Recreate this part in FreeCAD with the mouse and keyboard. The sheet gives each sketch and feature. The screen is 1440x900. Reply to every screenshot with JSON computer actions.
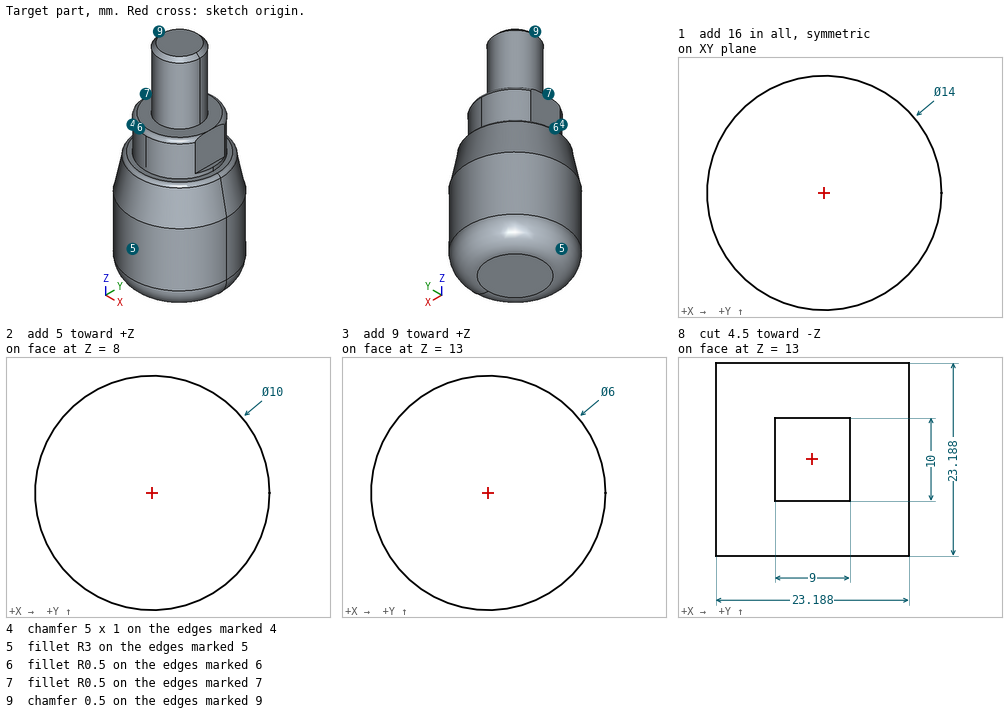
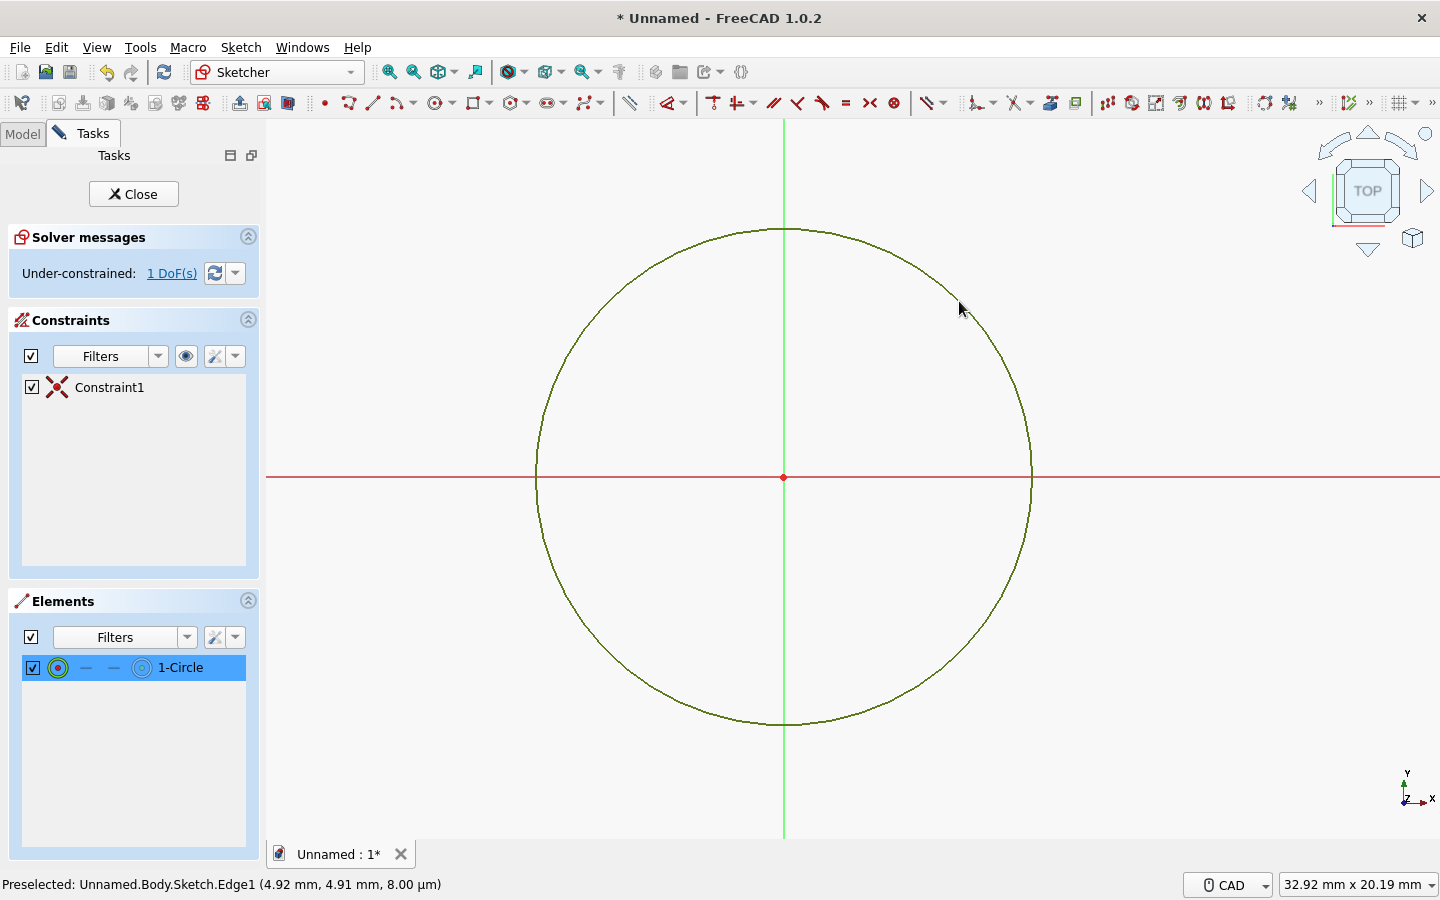
{"action": "key", "text": "k o"}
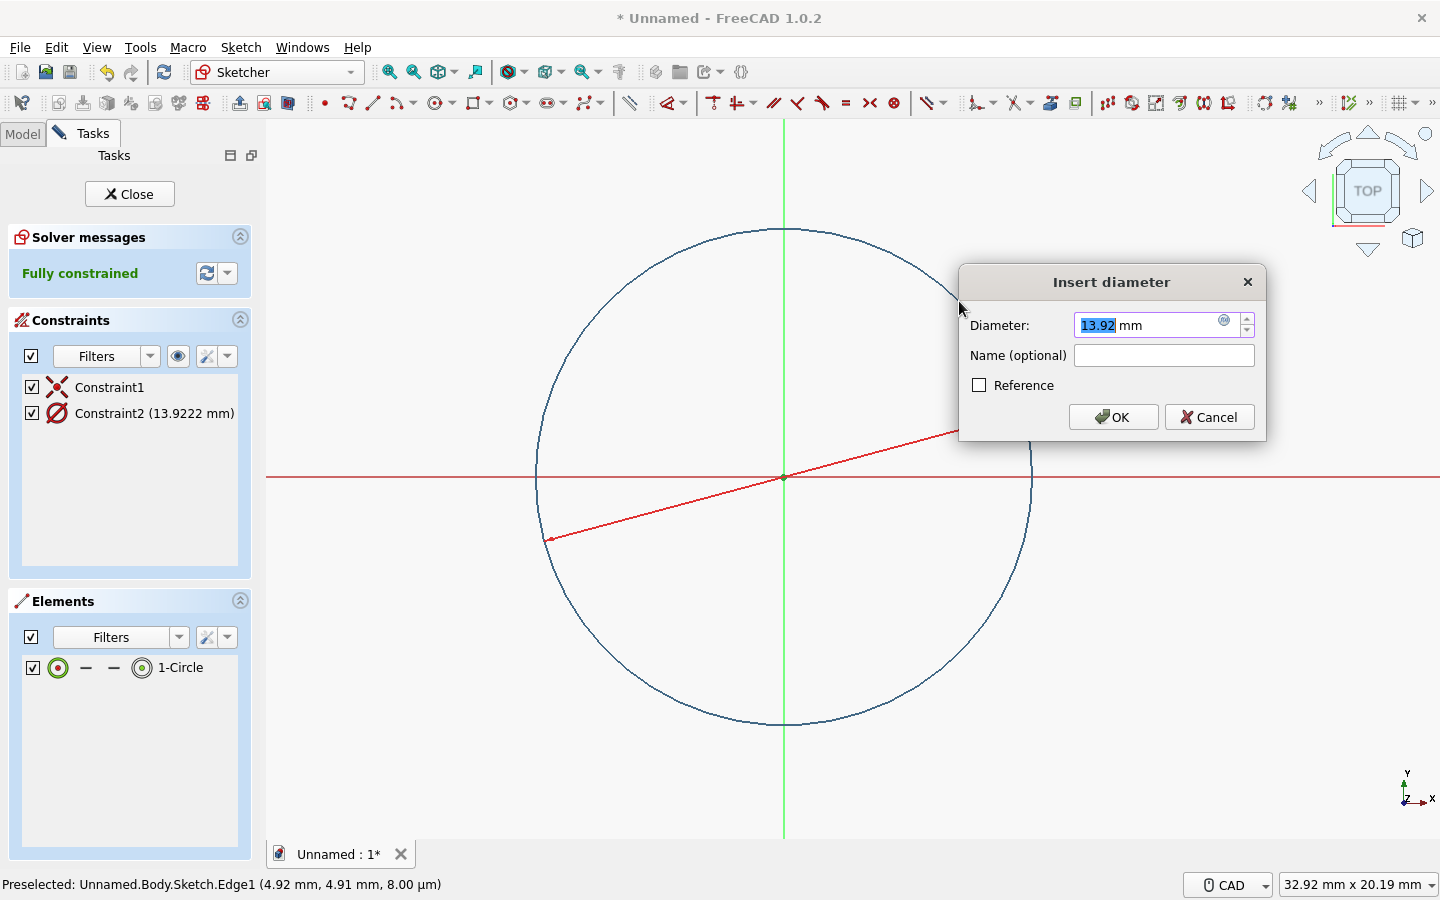
{"action": "type", "text": "14"}
{"action": "key", "text": "Return"}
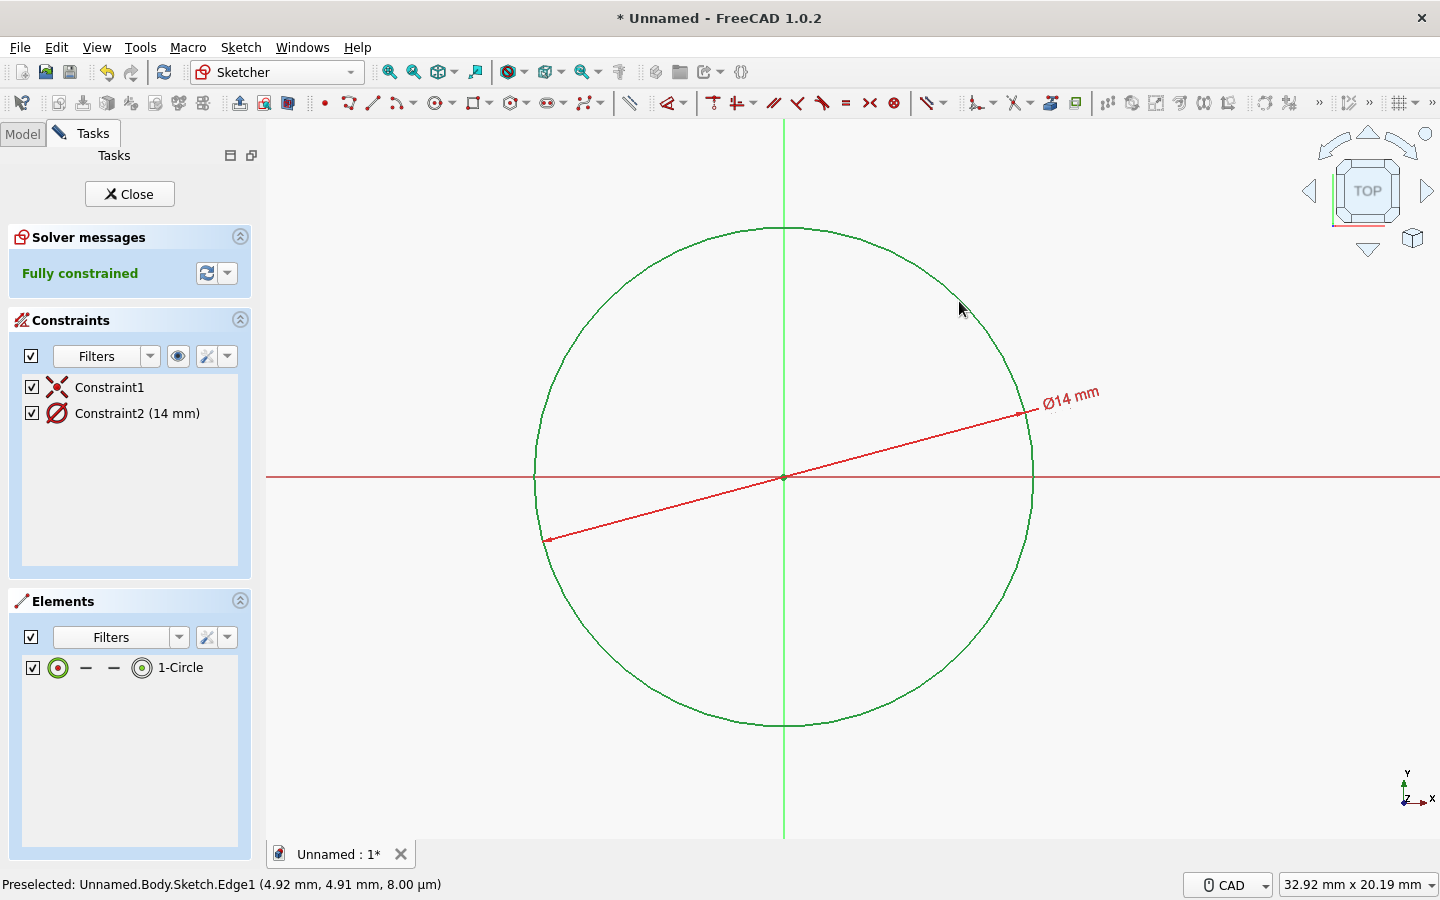
{"action": "left_click", "coordinate": [130, 194]}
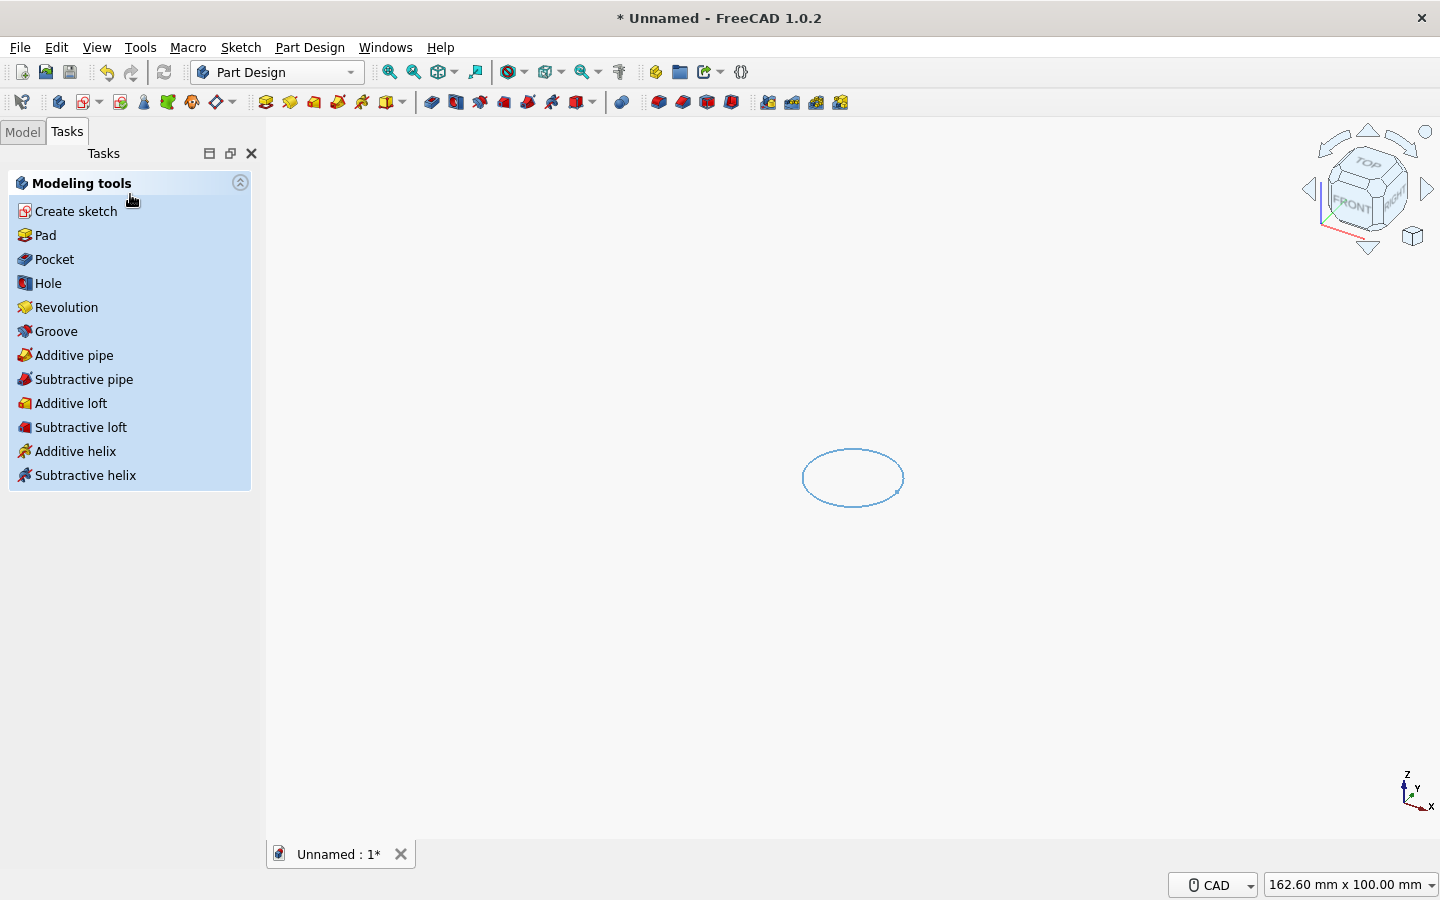
{"action": "left_click", "coordinate": [266, 102]}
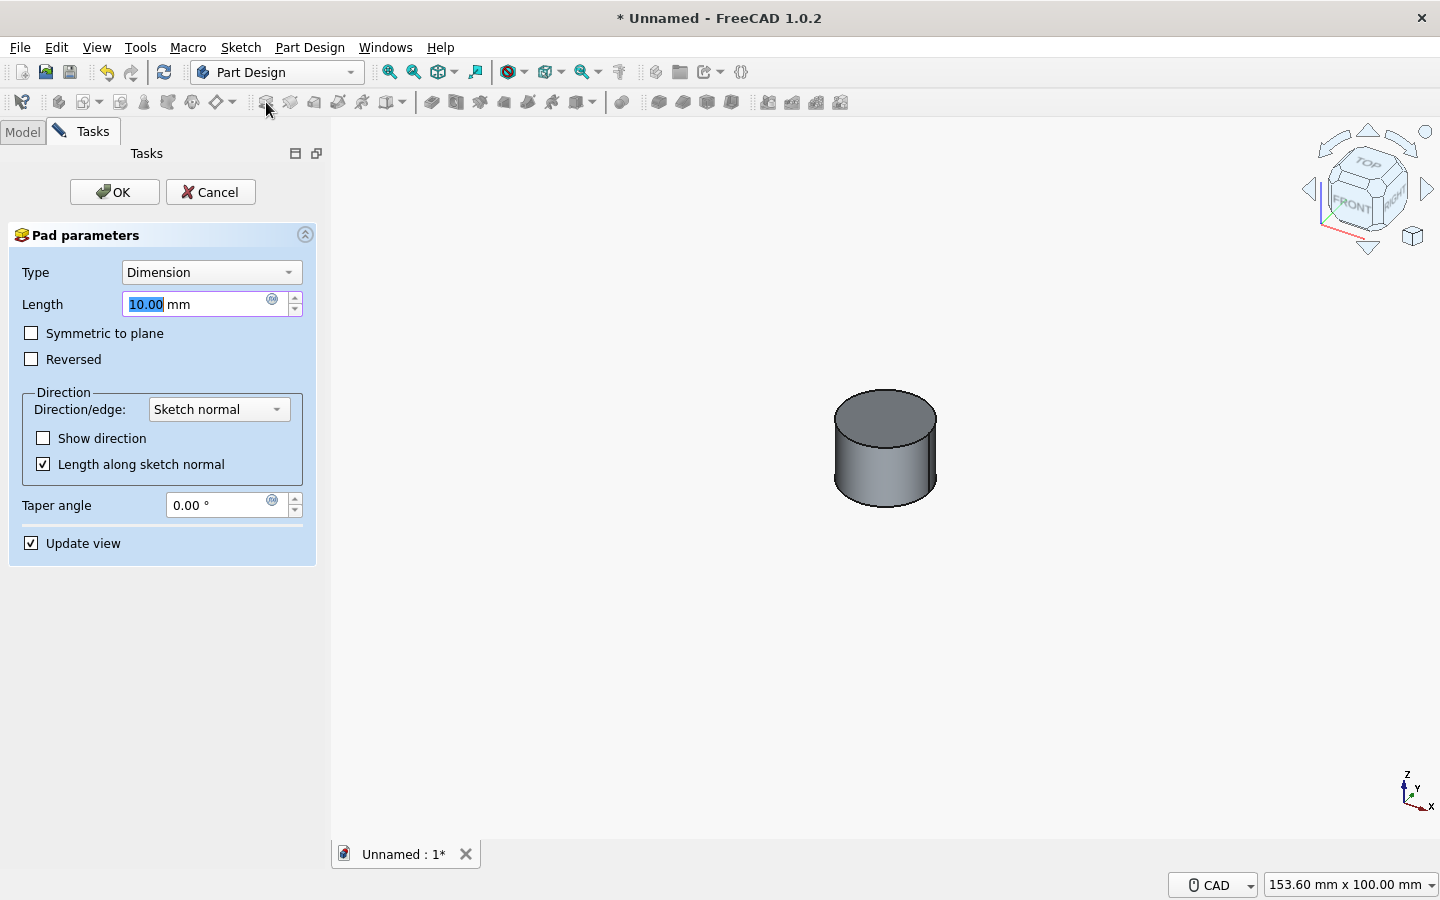
{"action": "type", "text": "16"}
{"action": "key", "text": "Tab"}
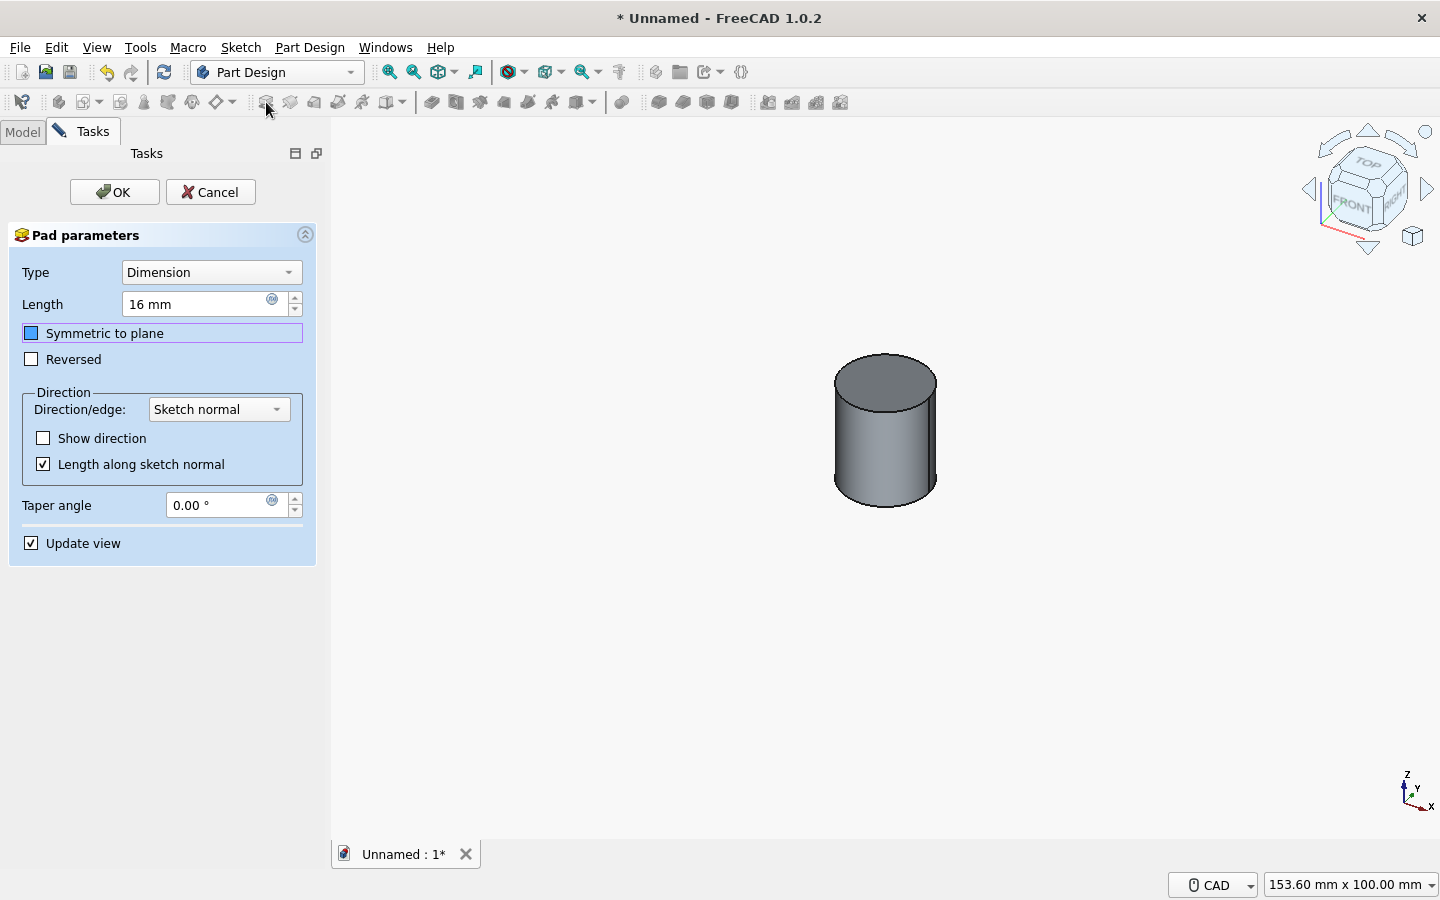
{"action": "left_click", "coordinate": [30, 333]}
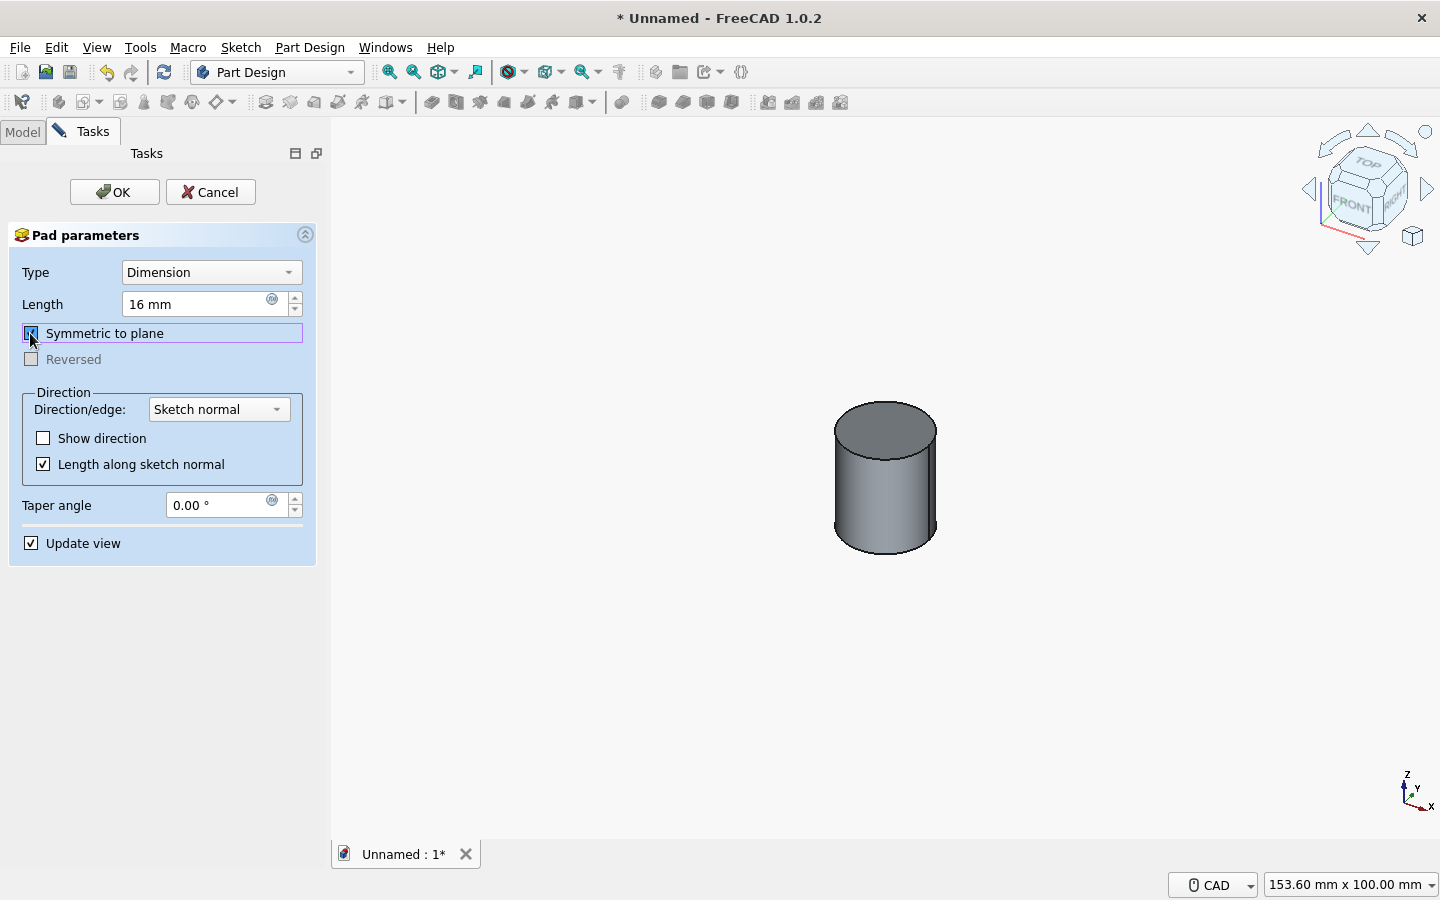
{"action": "left_click", "coordinate": [115, 192]}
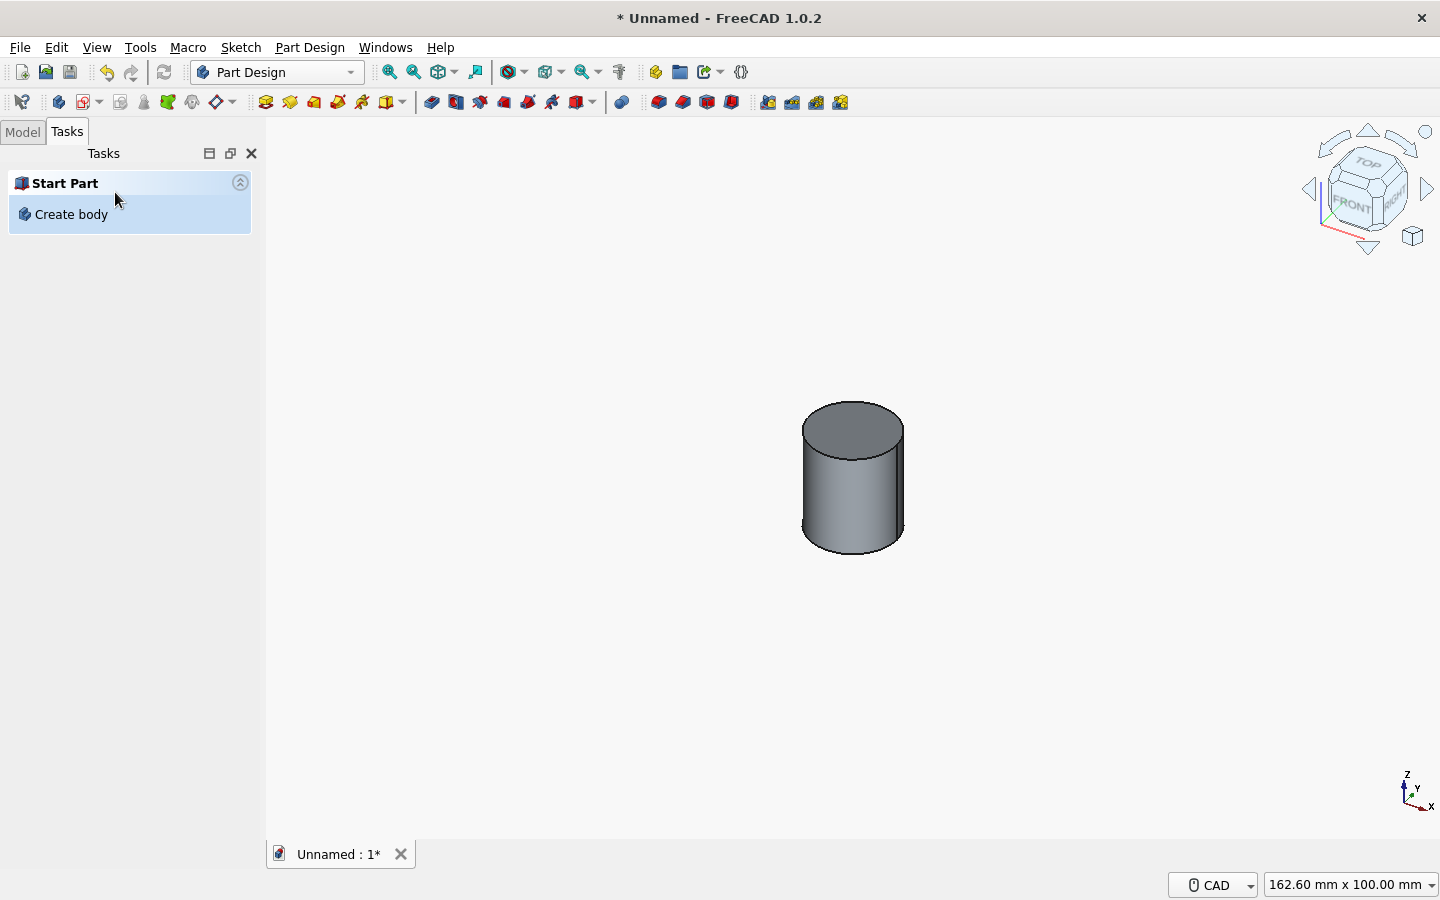
{"action": "key", "text": "v f"}